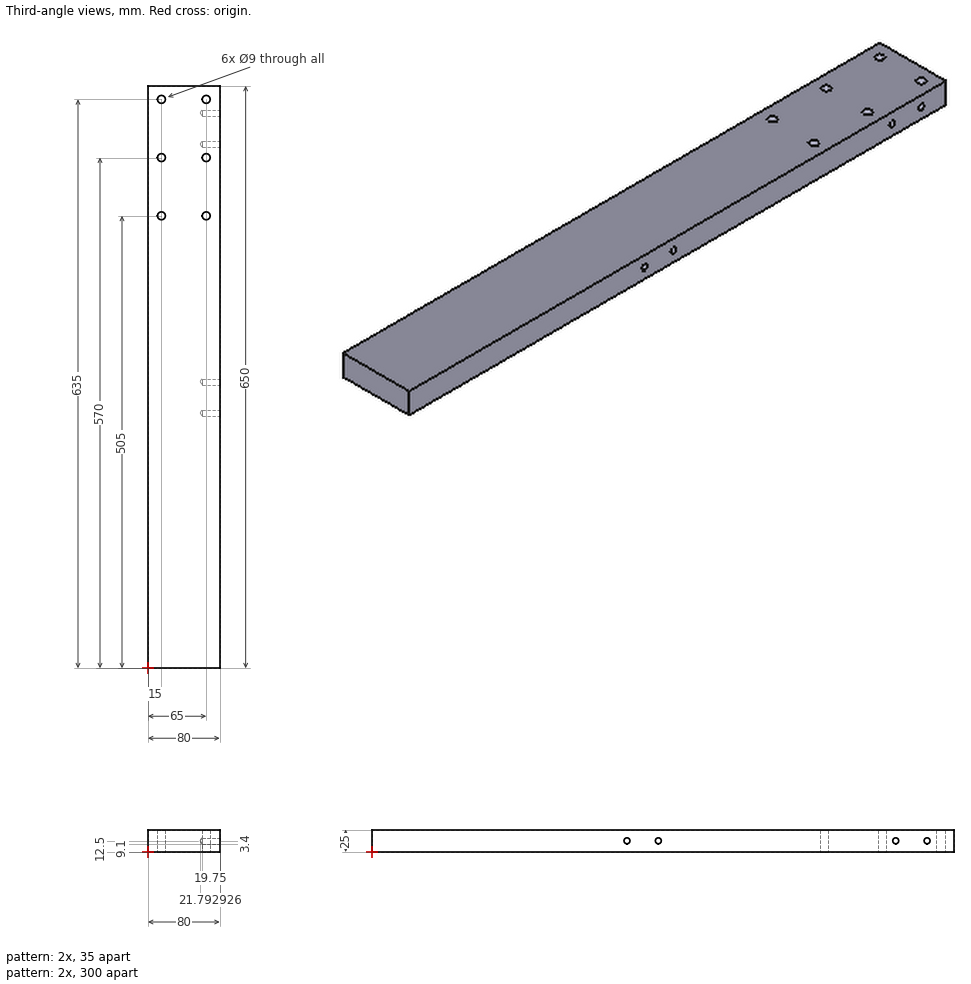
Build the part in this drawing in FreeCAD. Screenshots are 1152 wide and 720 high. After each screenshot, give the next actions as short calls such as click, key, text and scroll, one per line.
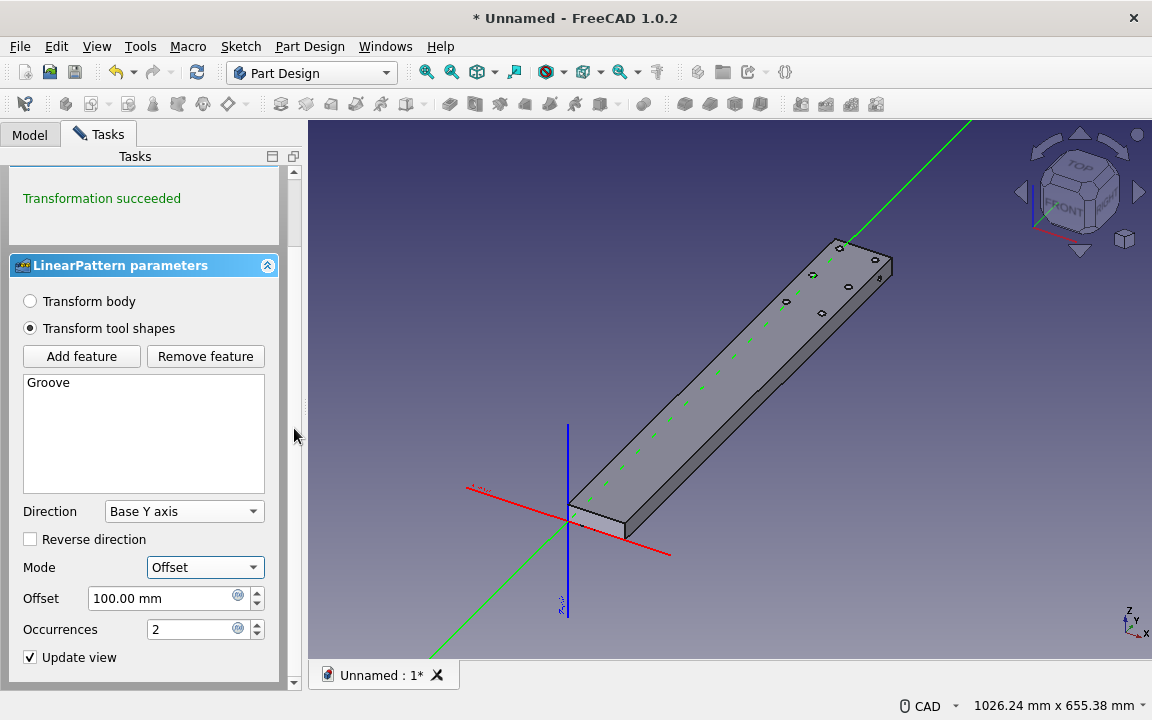
triple_click(170, 598)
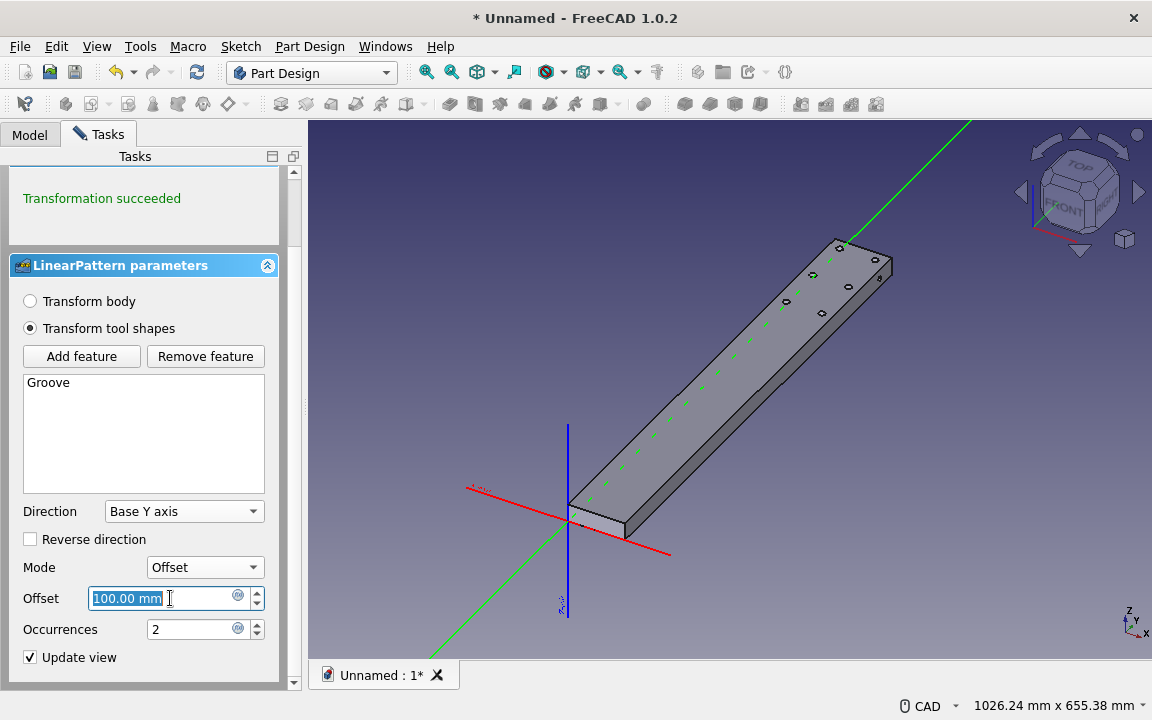
text(35)
key(Tab)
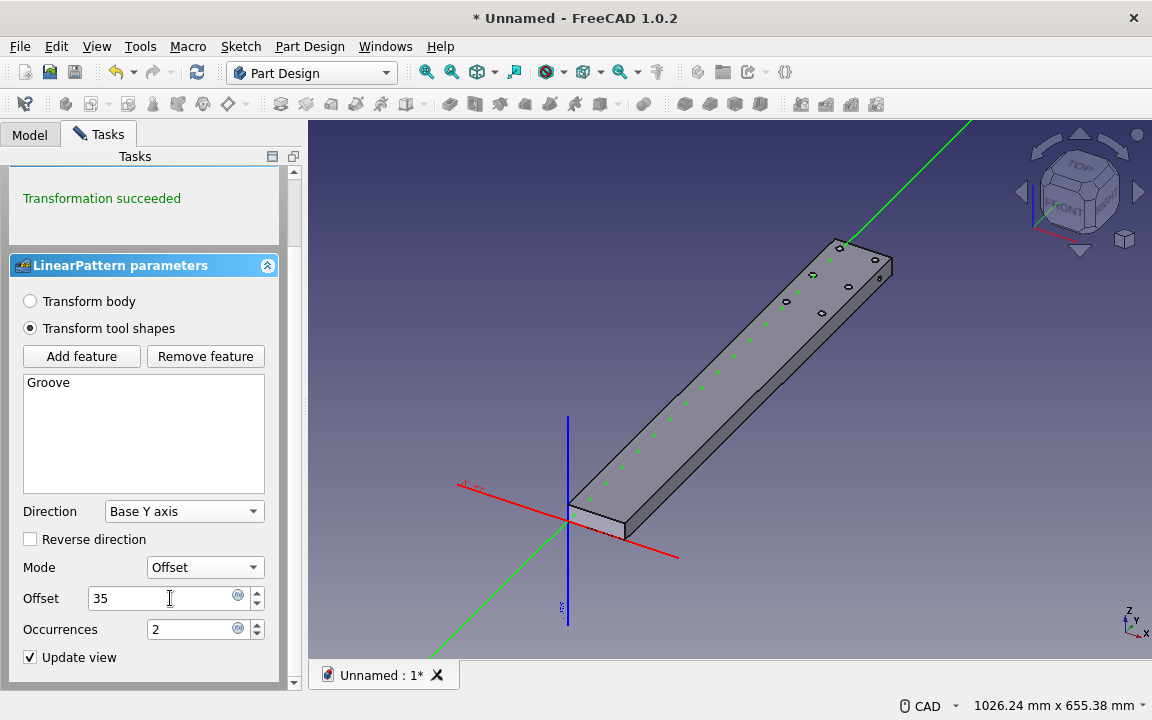
triple_click(199, 630)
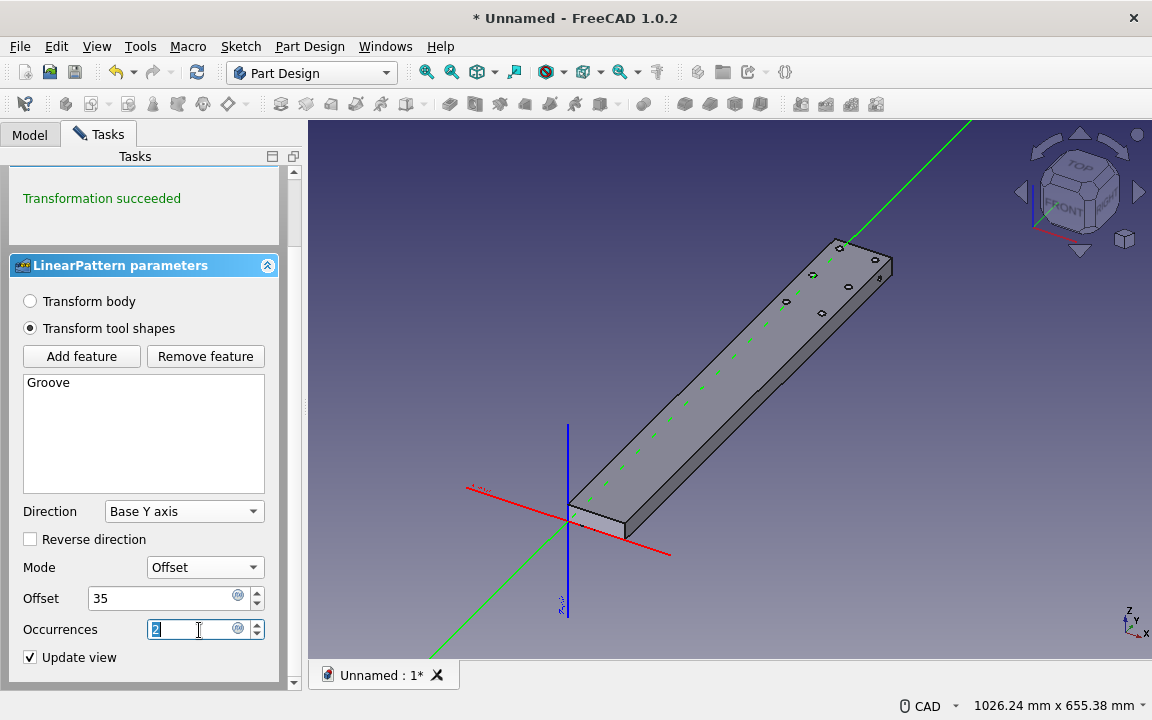
text(2)
key(Tab)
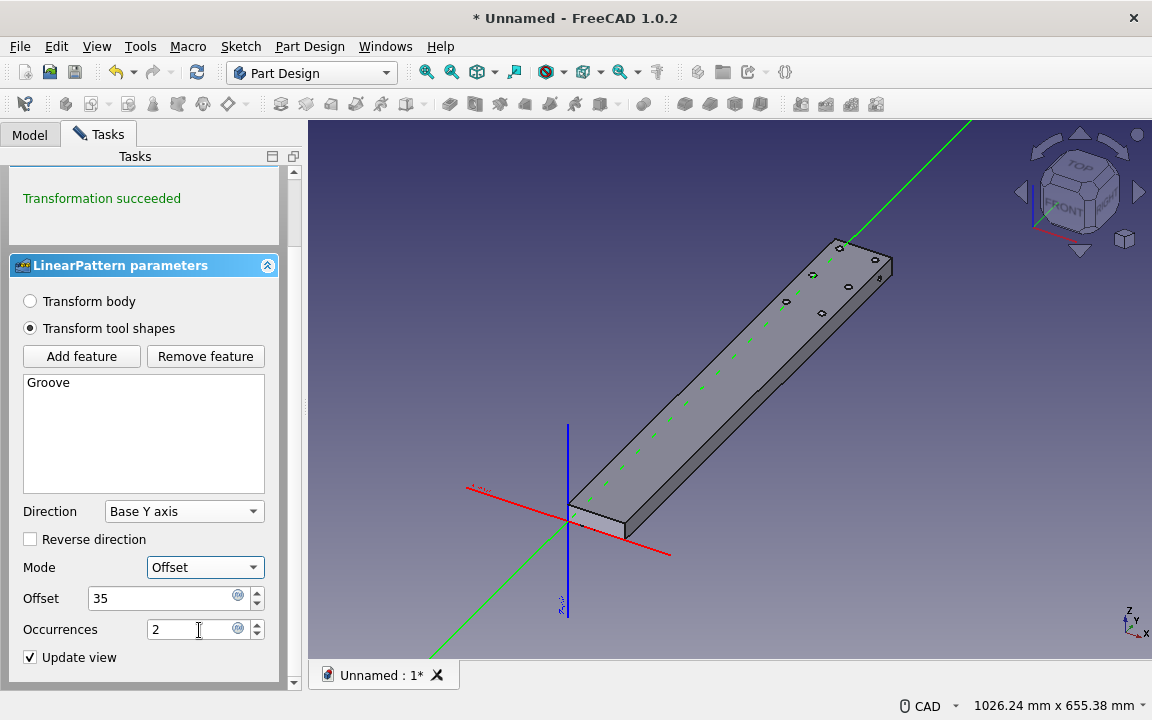
click(31, 539)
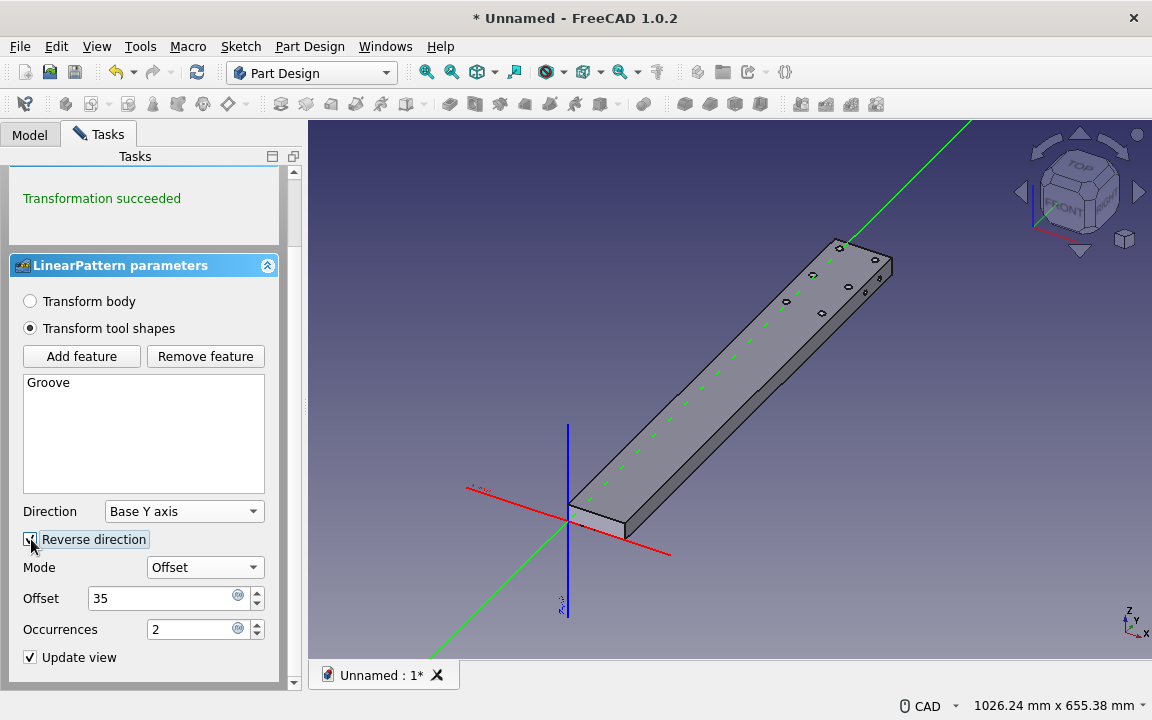
scroll(294, 428, up, 3)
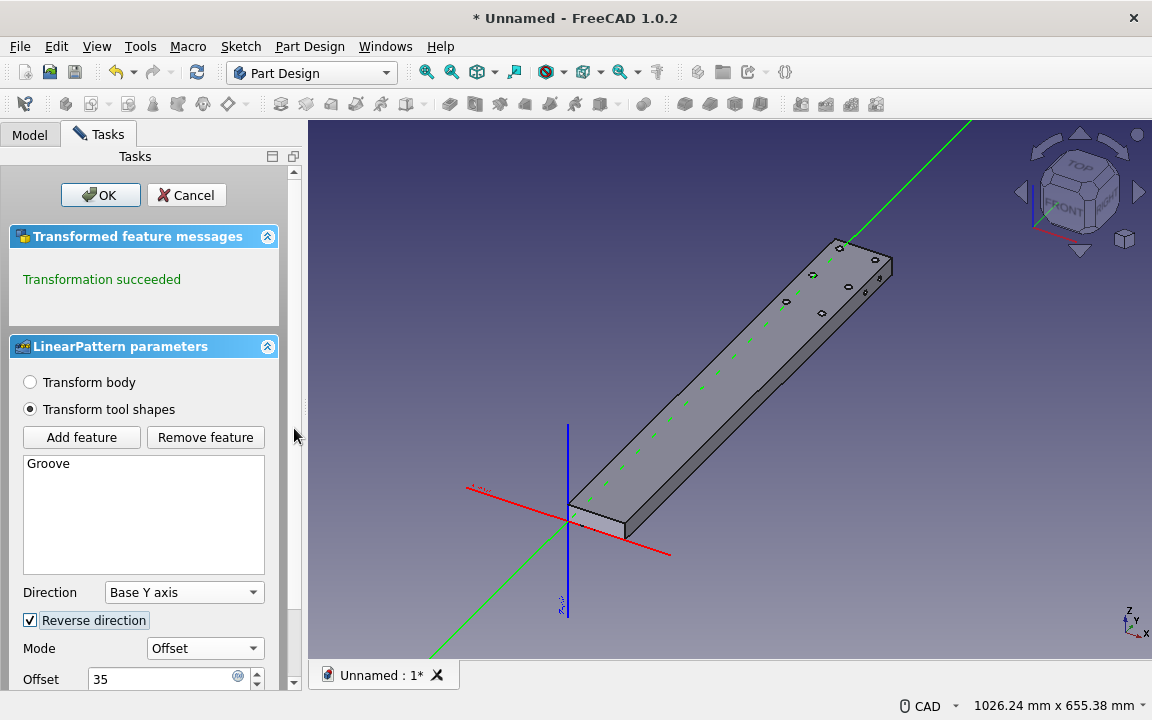
click(101, 195)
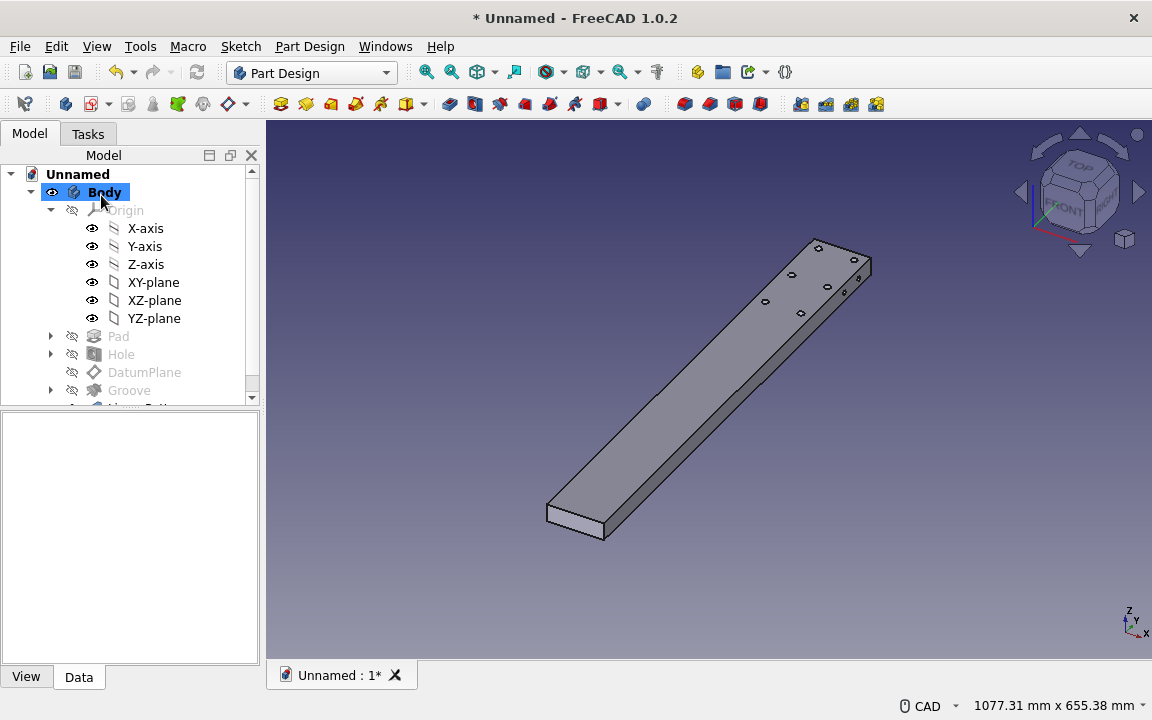
click(117, 390)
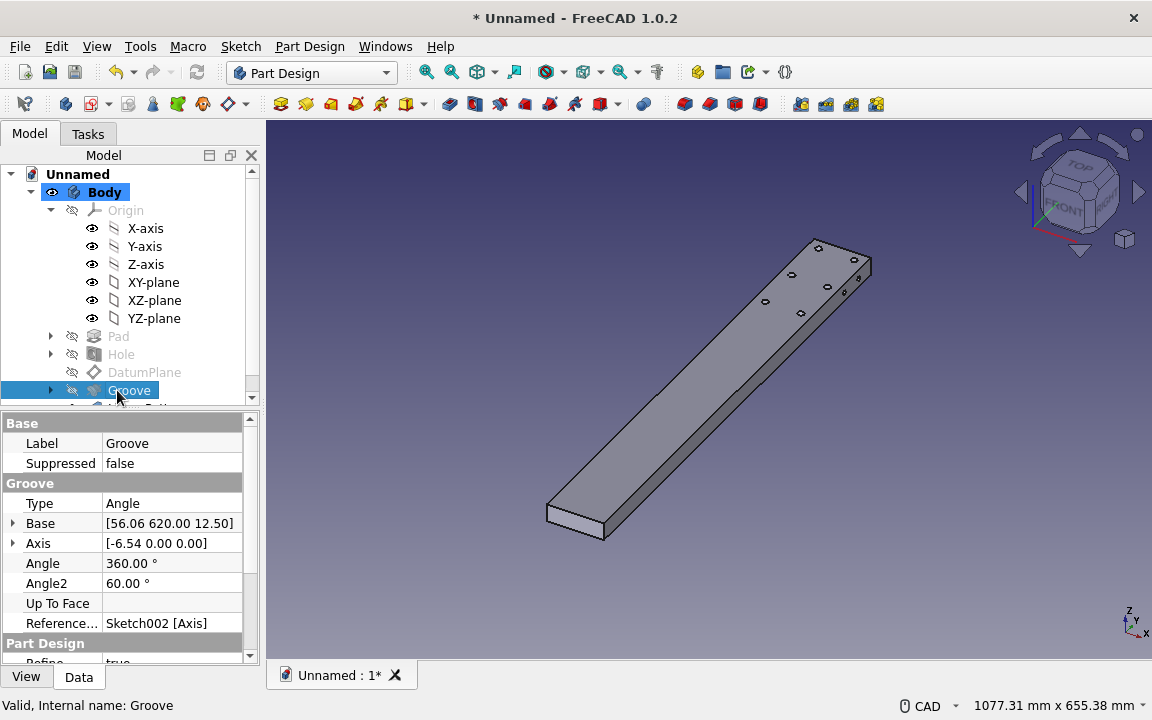
click(826, 104)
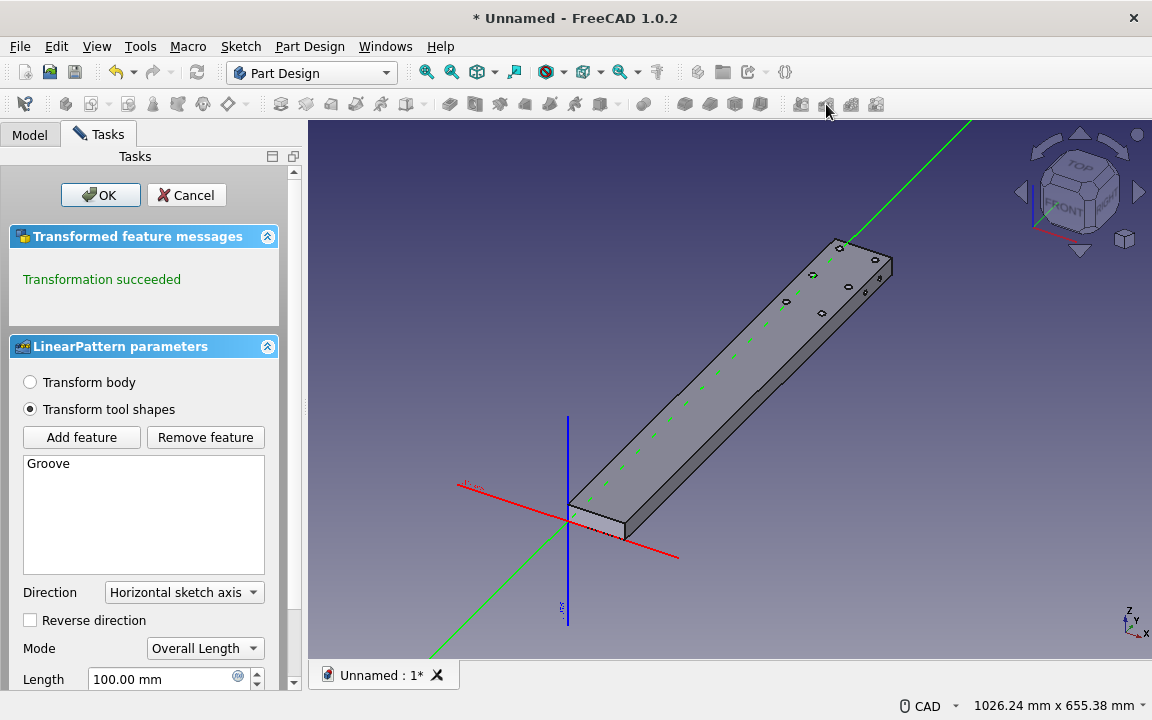
click(185, 592)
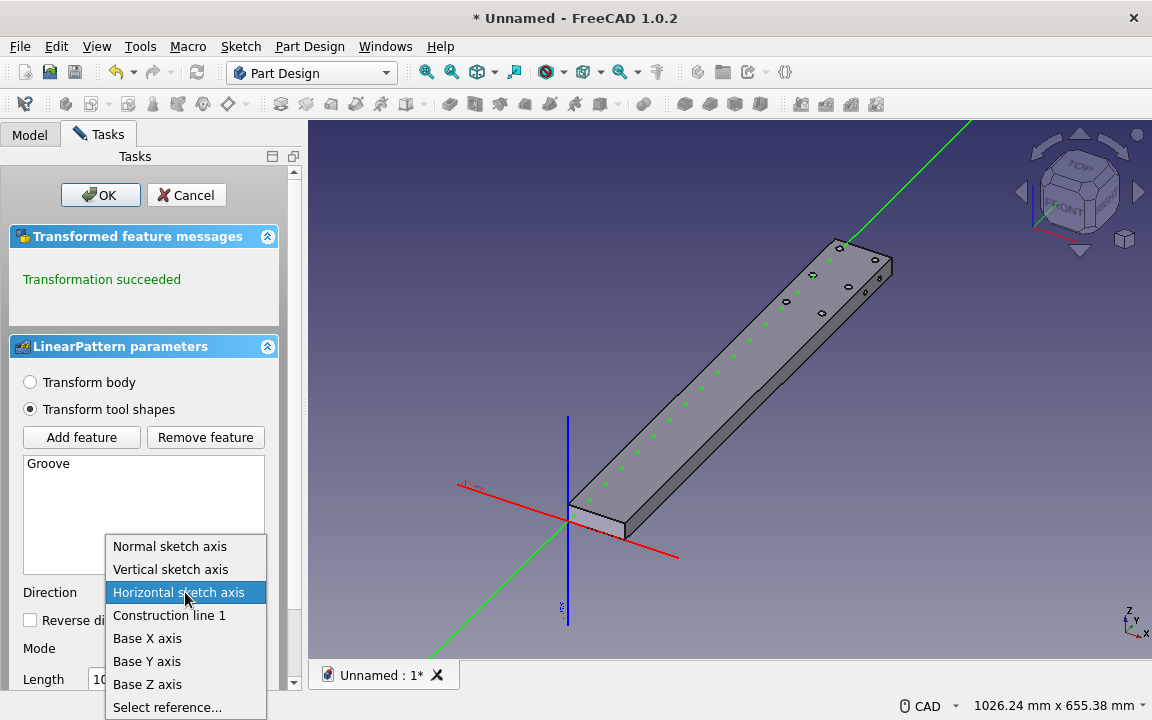
click(184, 662)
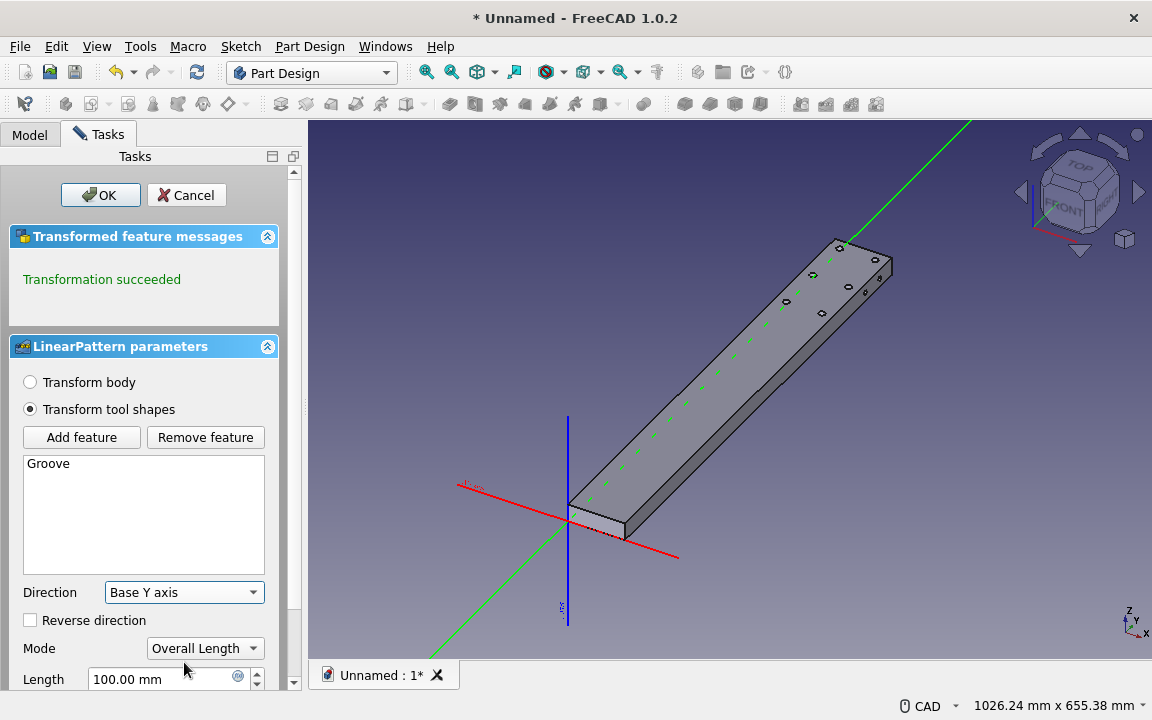
click(206, 648)